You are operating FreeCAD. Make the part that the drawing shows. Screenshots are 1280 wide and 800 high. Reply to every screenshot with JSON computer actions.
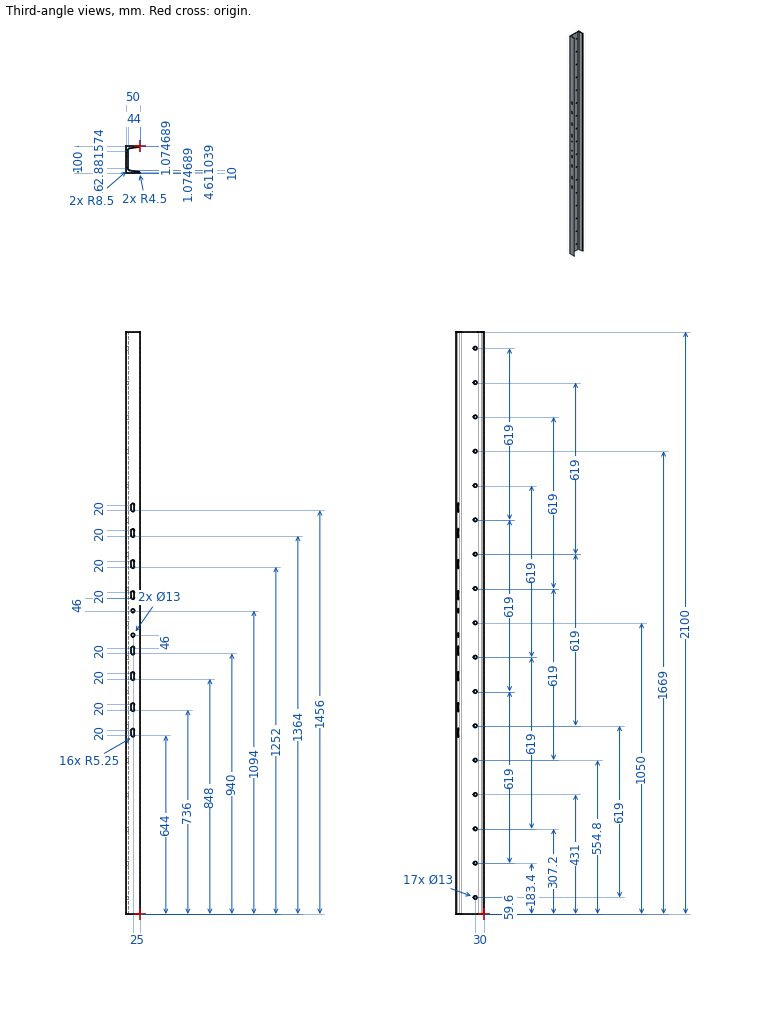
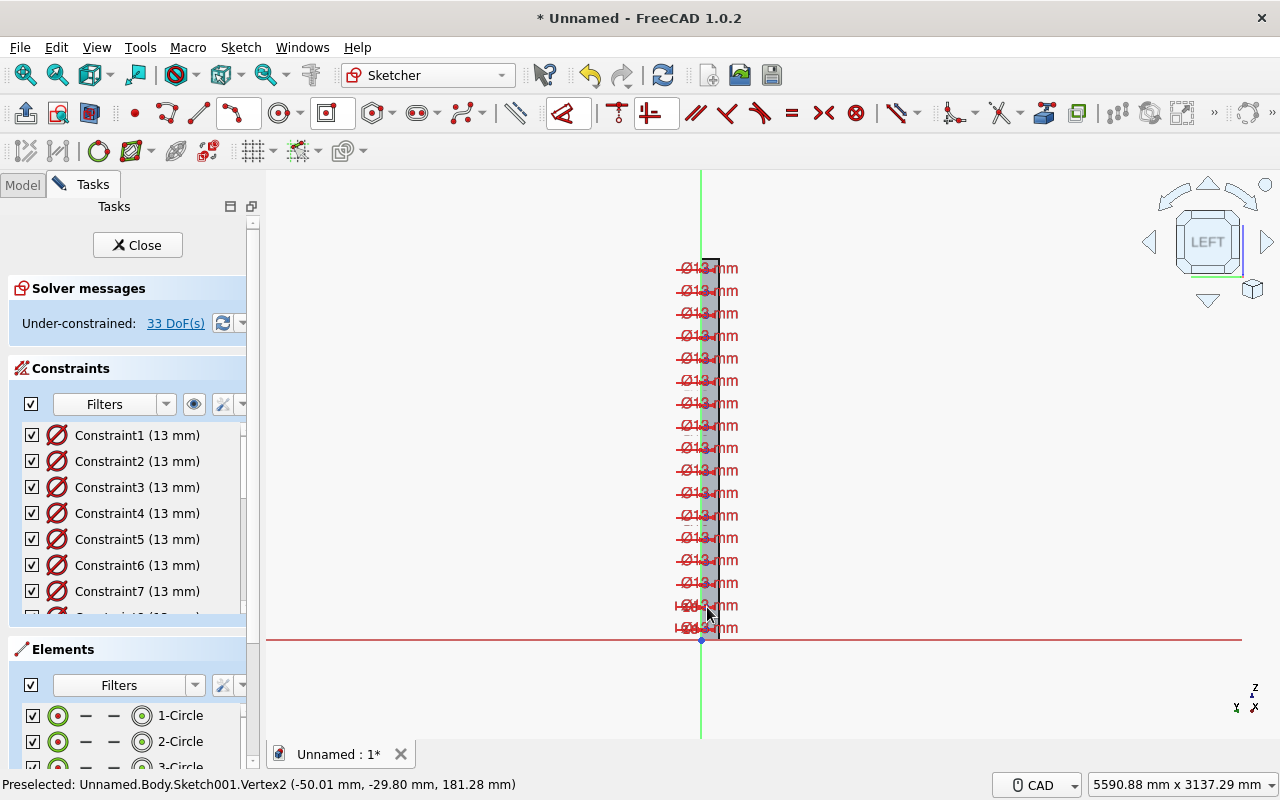
{"action": "left_click", "coordinate": [707, 607]}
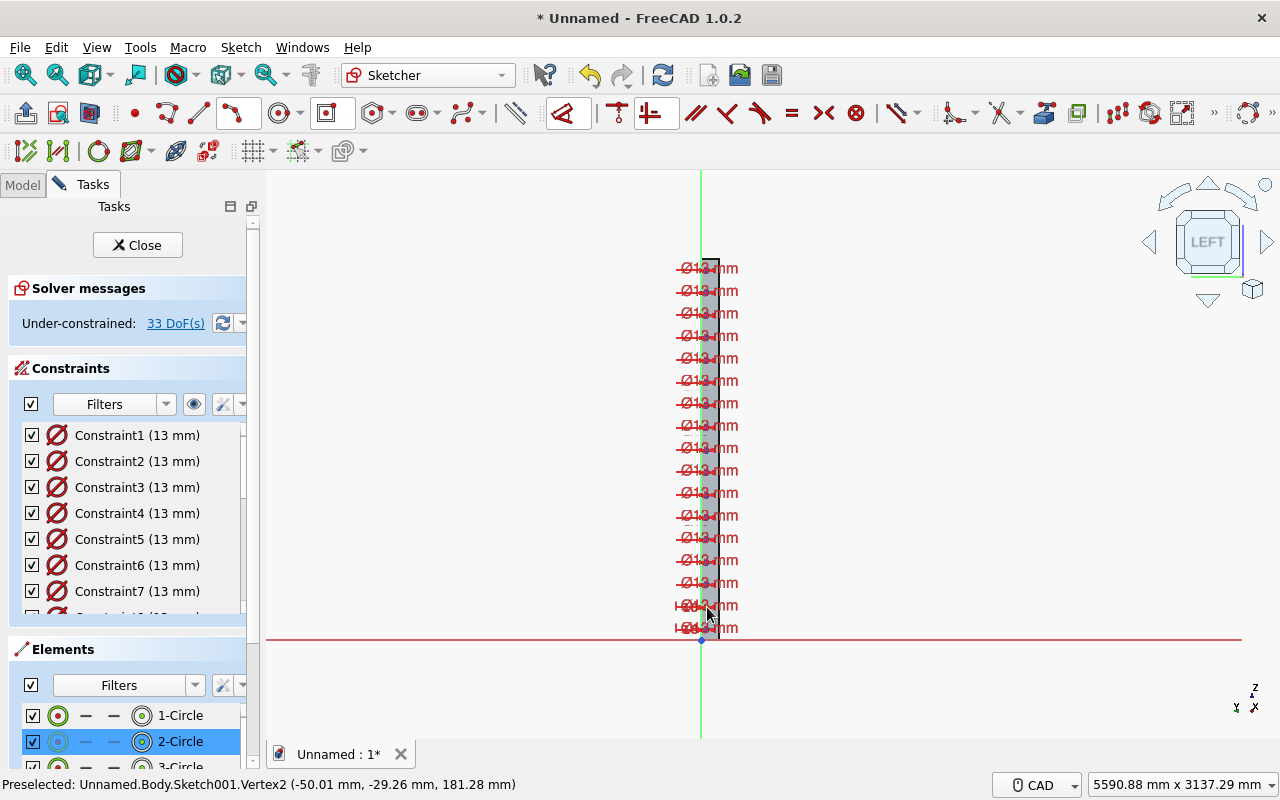
{"action": "left_click", "coordinate": [707, 585]}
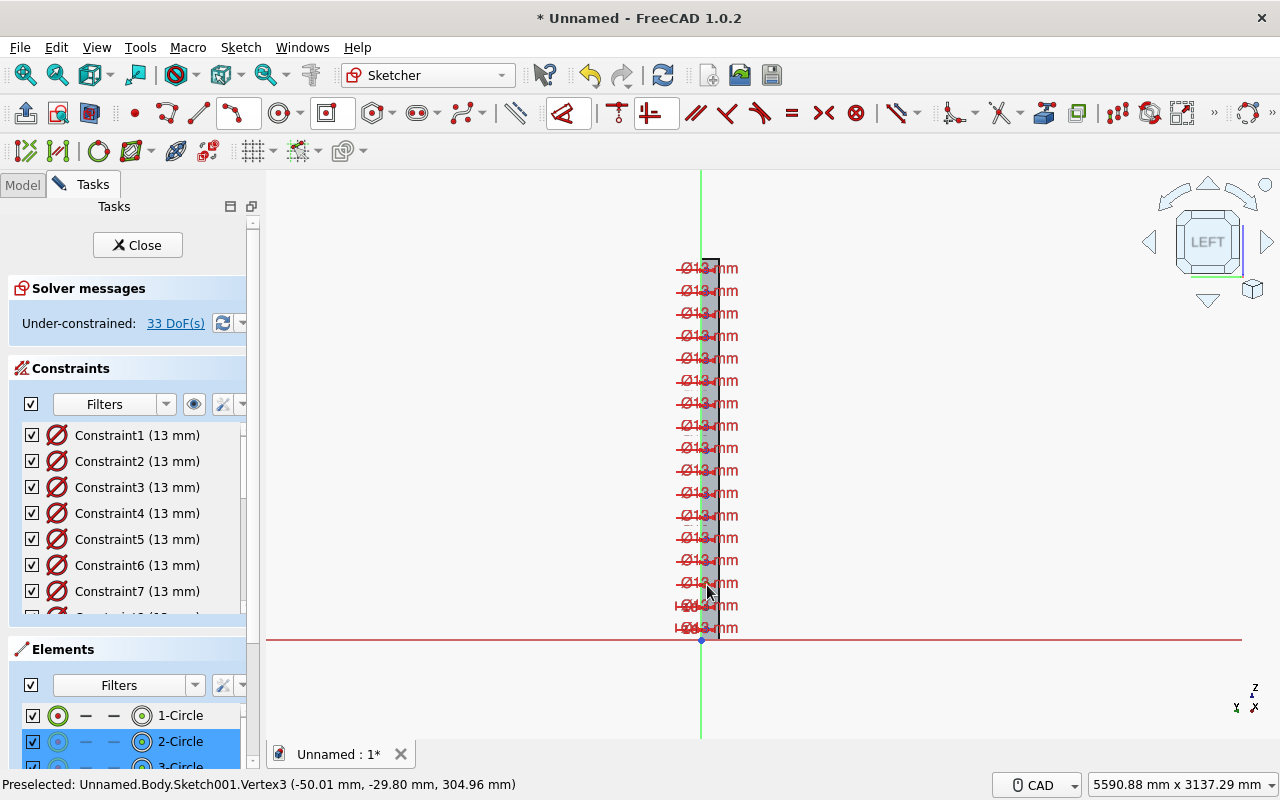
{"action": "key", "text": "v"}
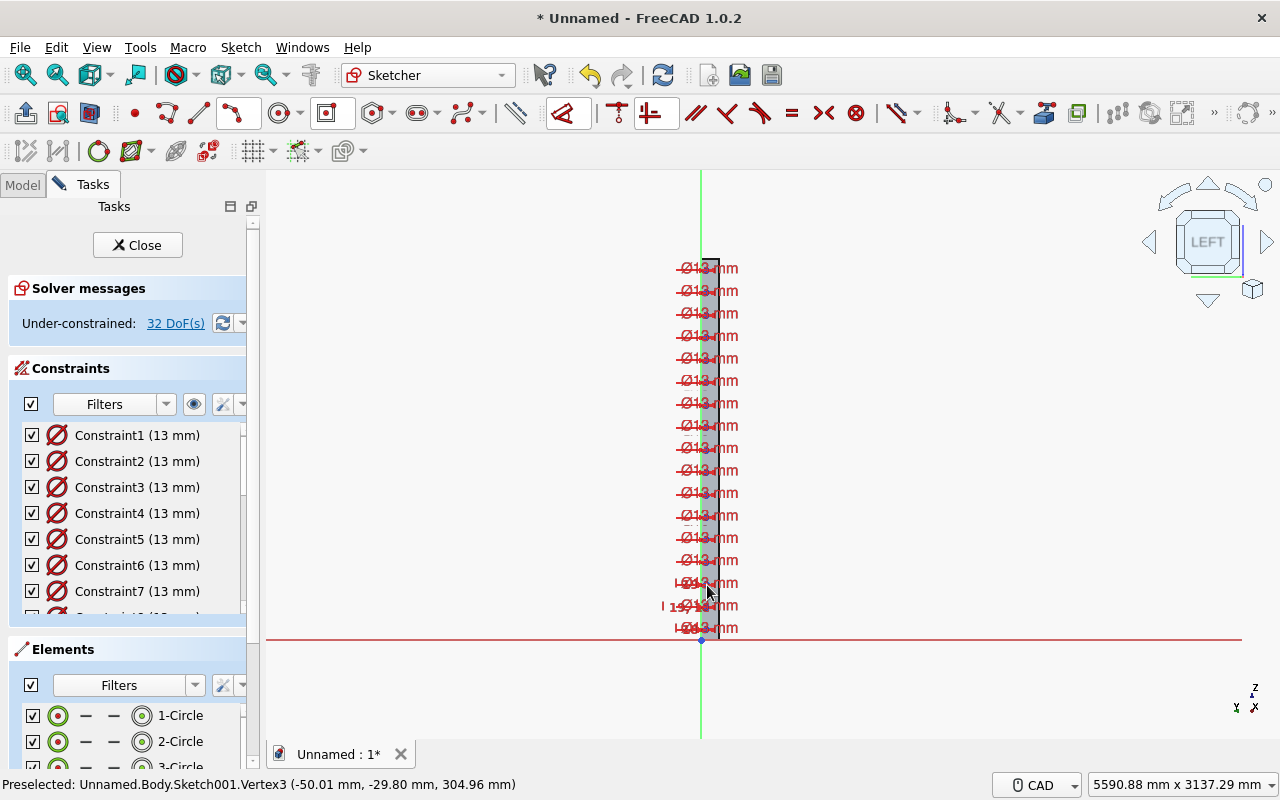
{"action": "left_click", "coordinate": [707, 585]}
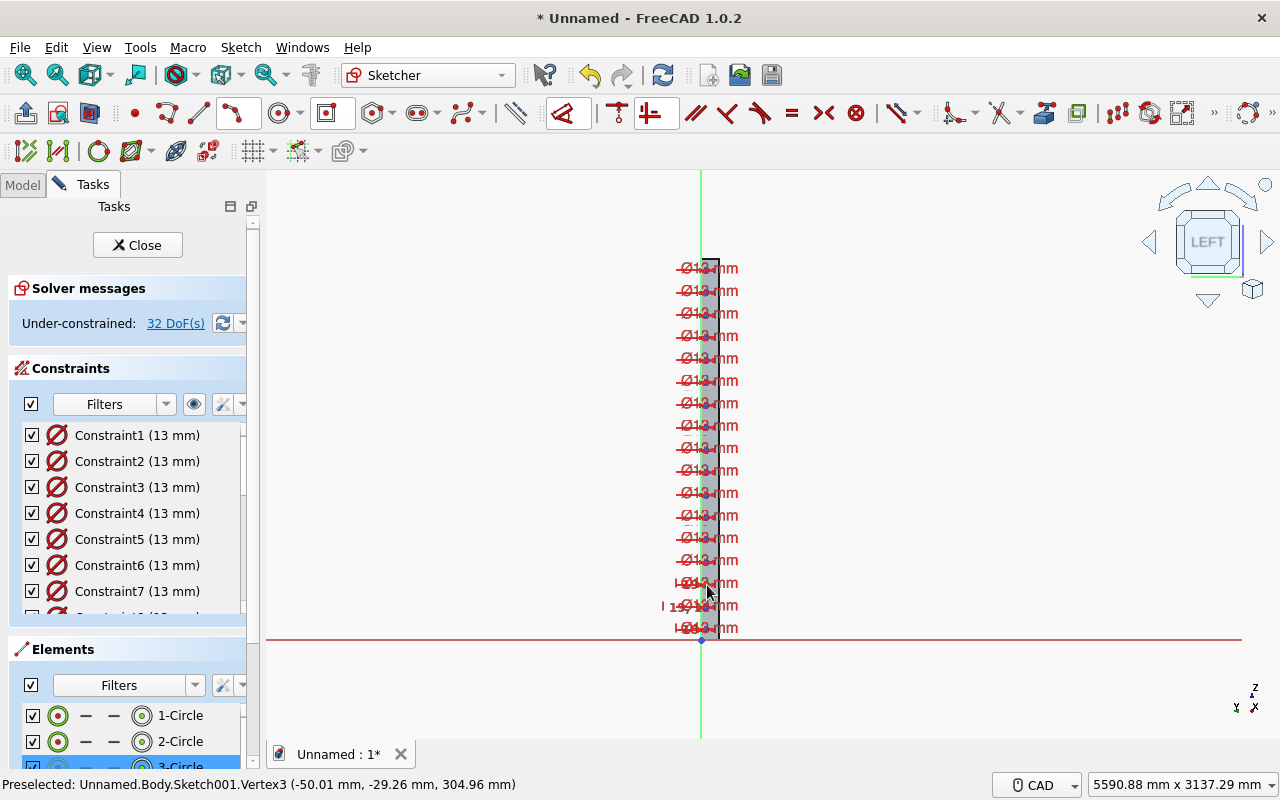
{"action": "left_click", "coordinate": [707, 562]}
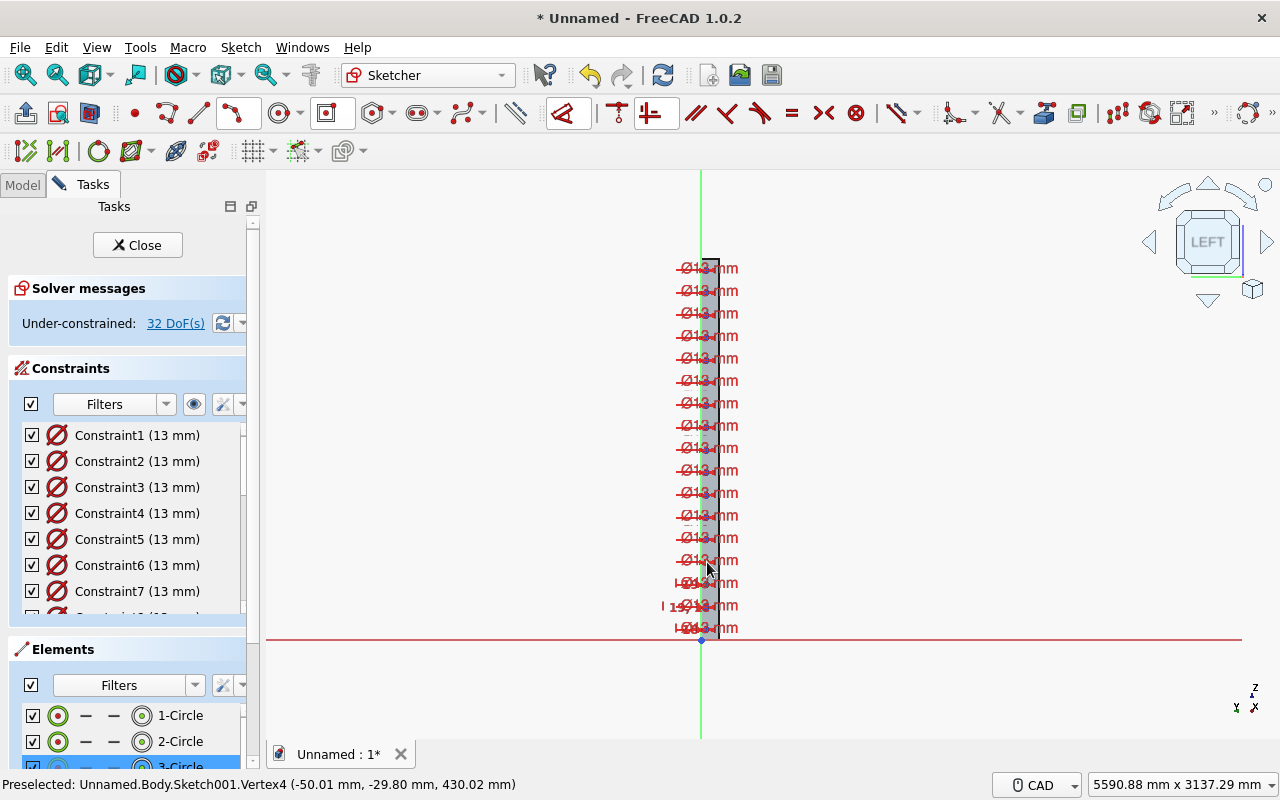
{"action": "key", "text": "v"}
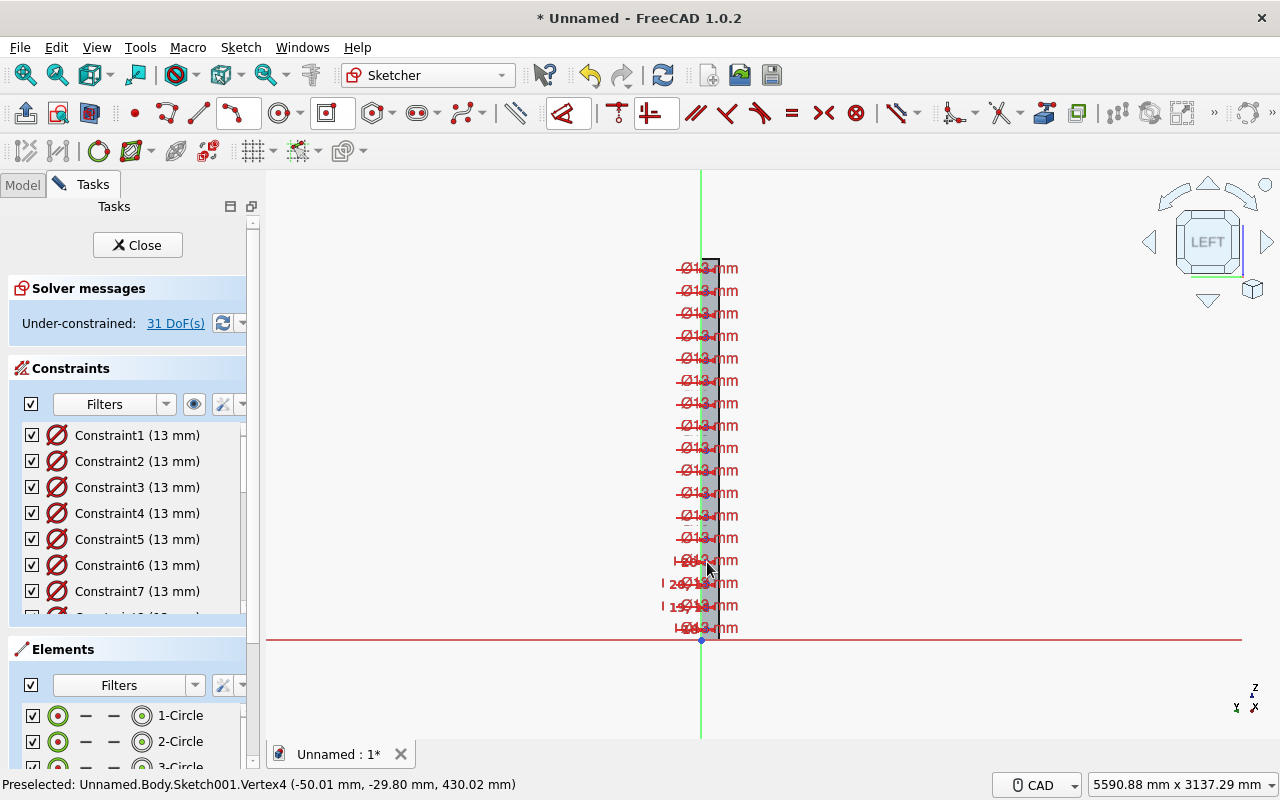
{"action": "left_click", "coordinate": [707, 562]}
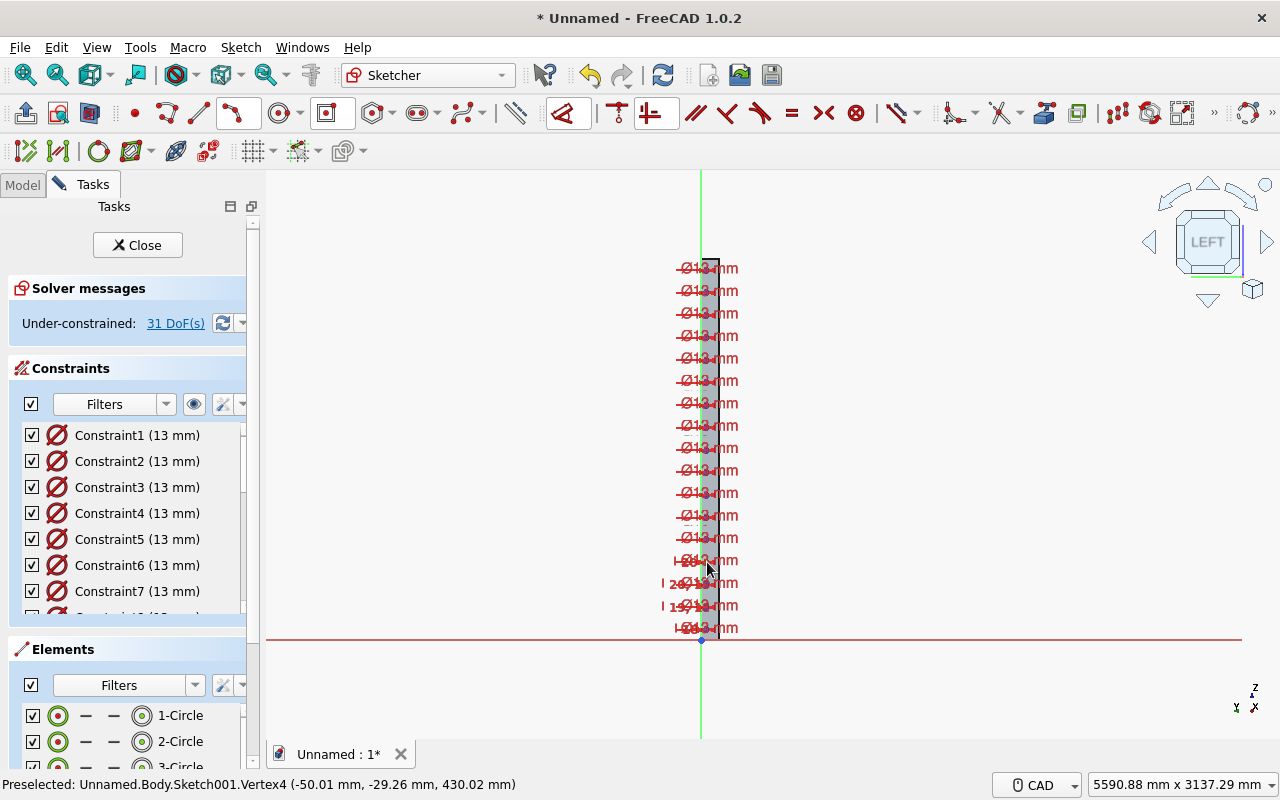
{"action": "left_click", "coordinate": [707, 540]}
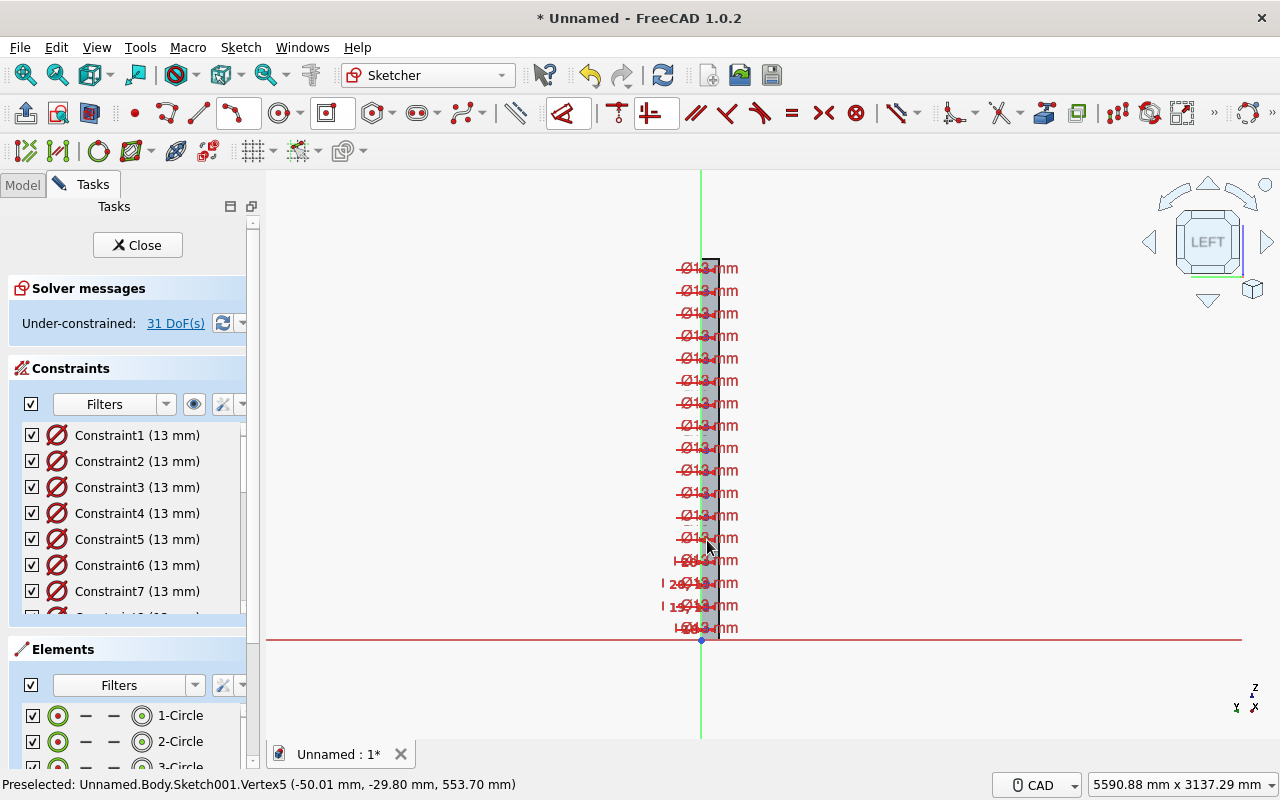
{"action": "left_click", "coordinate": [674, 114]}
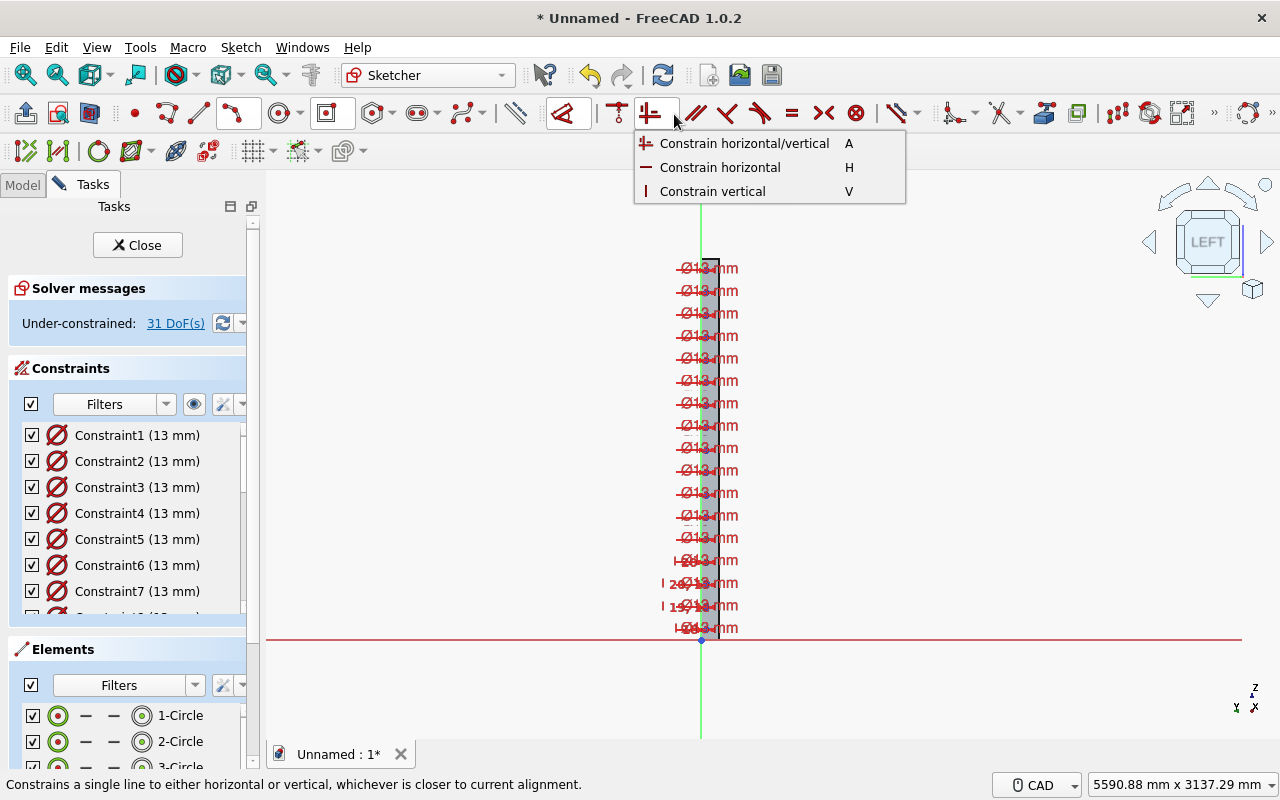
{"action": "left_click", "coordinate": [770, 191]}